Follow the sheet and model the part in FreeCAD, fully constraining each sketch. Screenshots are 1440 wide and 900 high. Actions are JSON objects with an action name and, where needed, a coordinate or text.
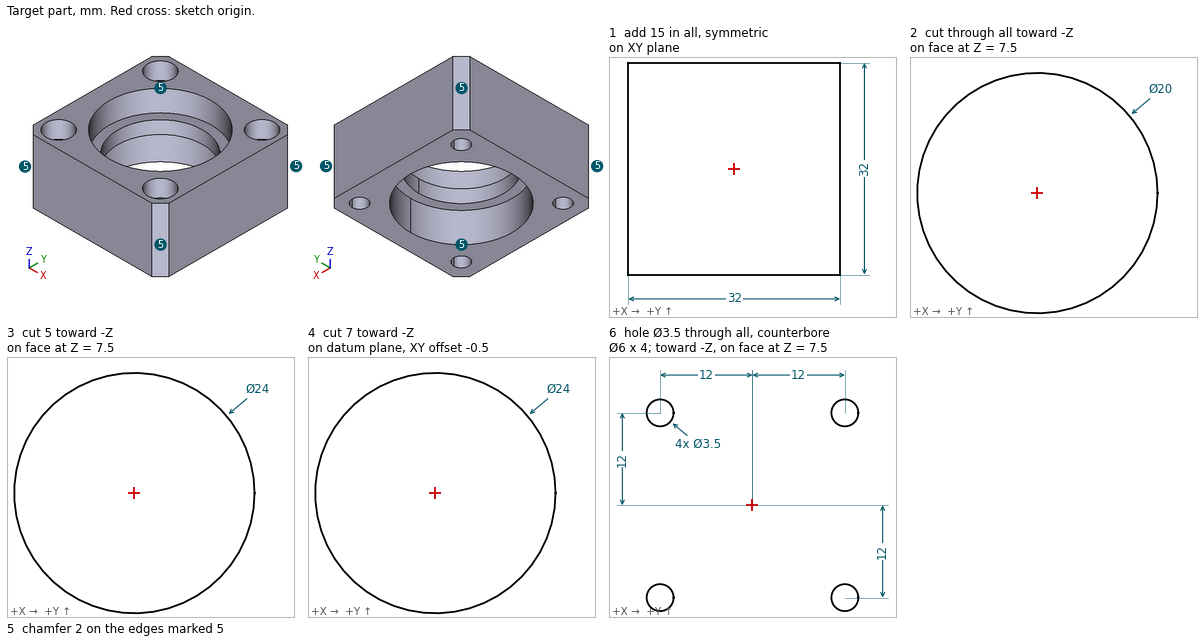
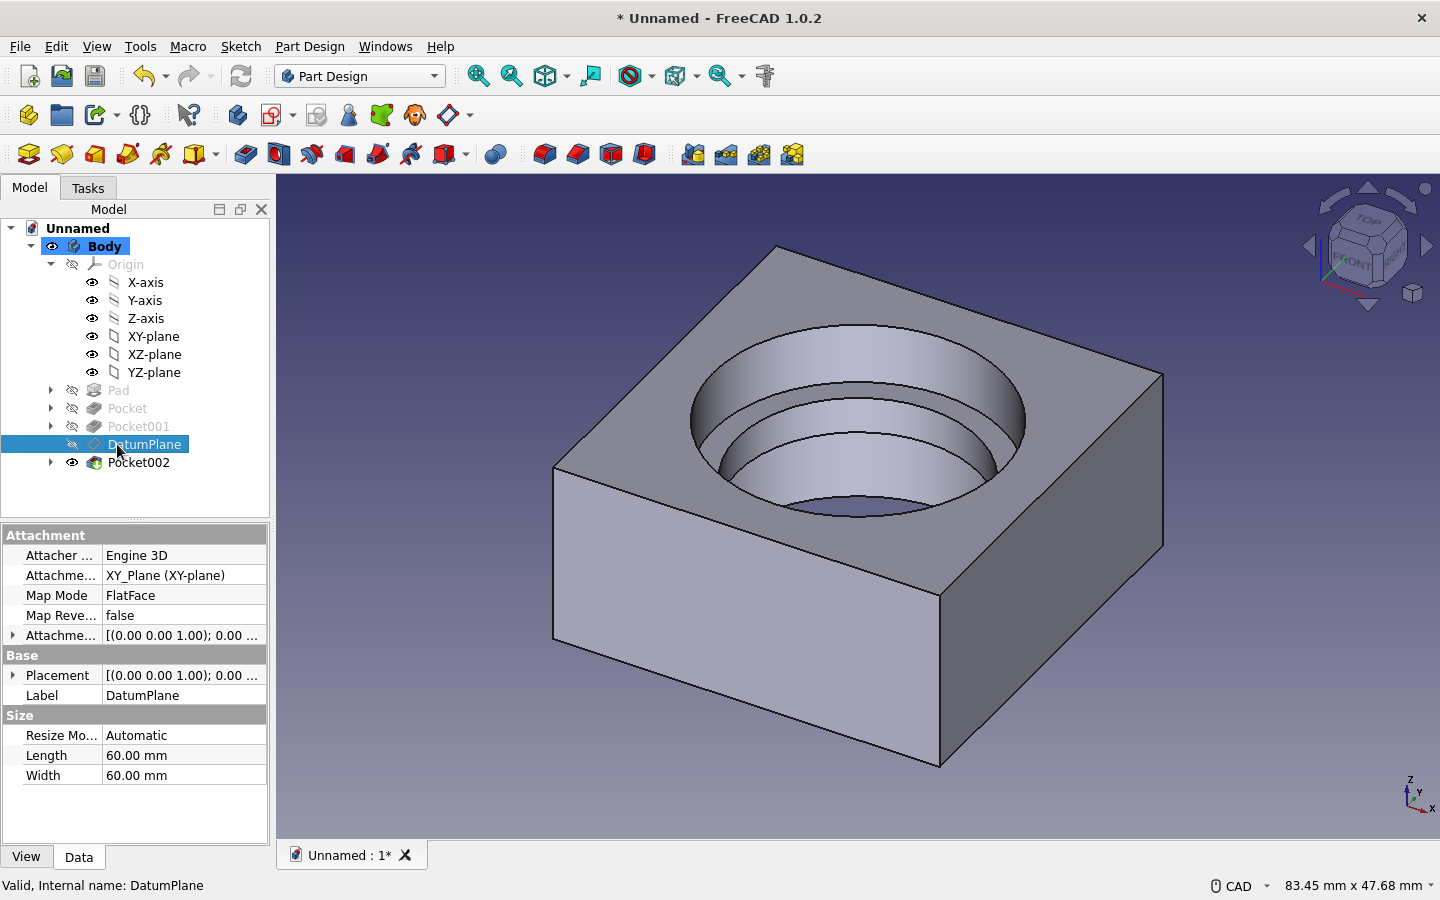
{"action": "left_click", "coordinate": [940, 680]}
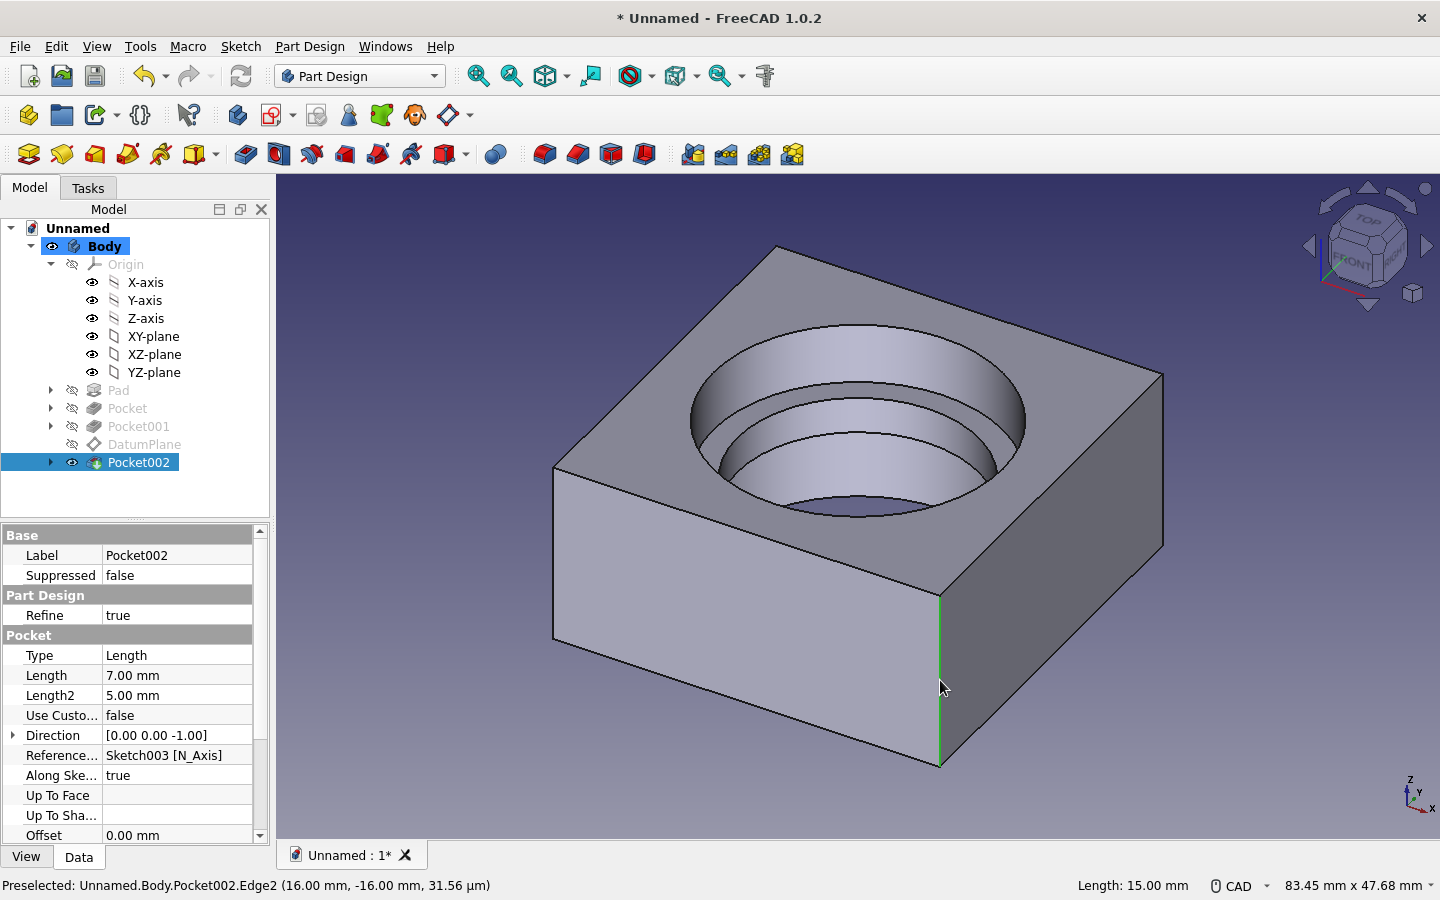
{"action": "key", "text": "0"}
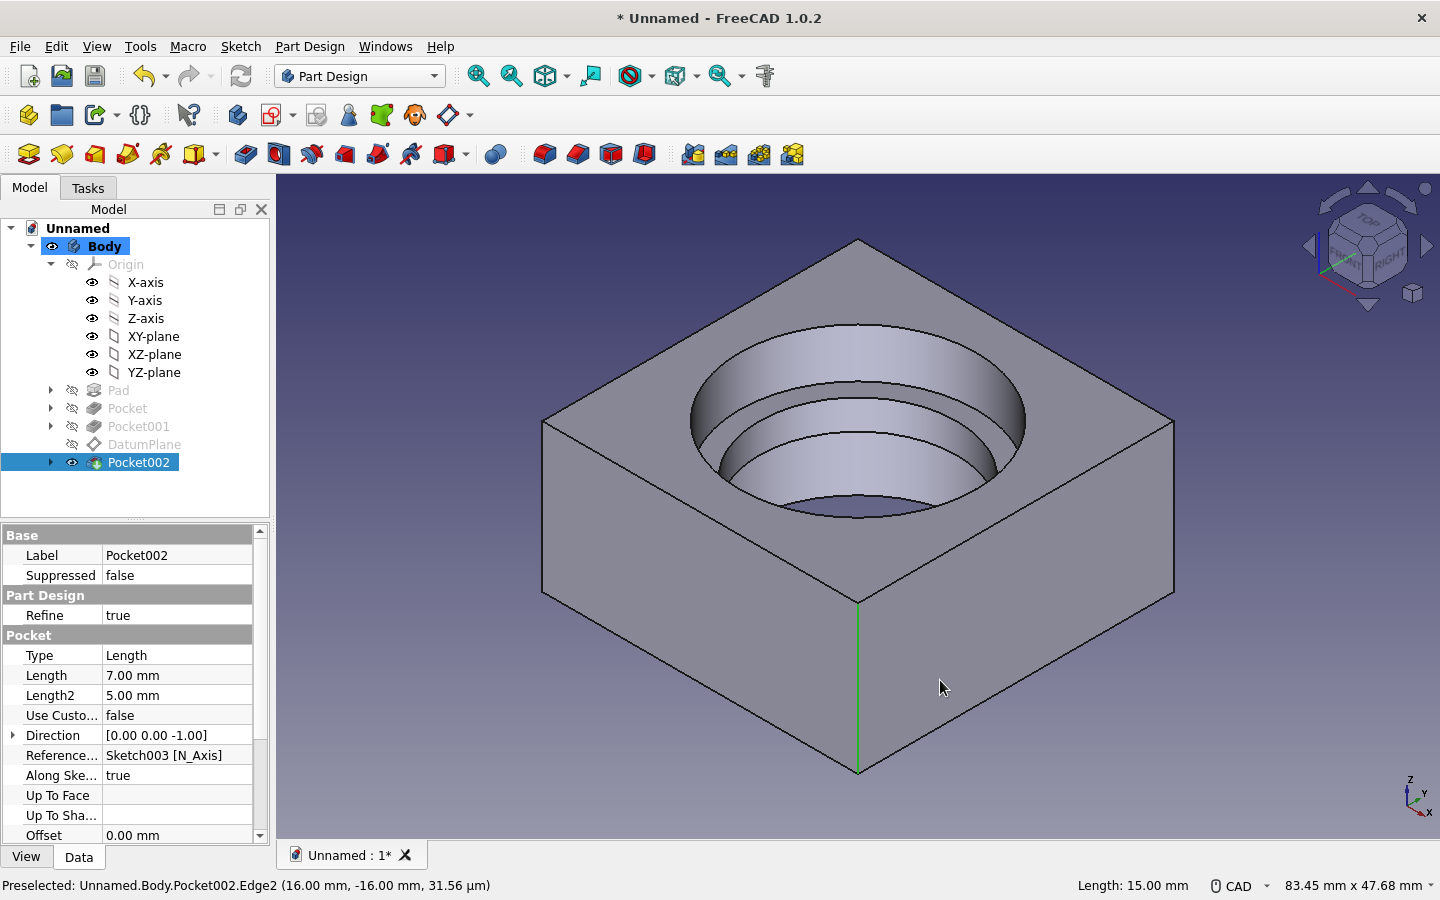
{"action": "key", "text": "2"}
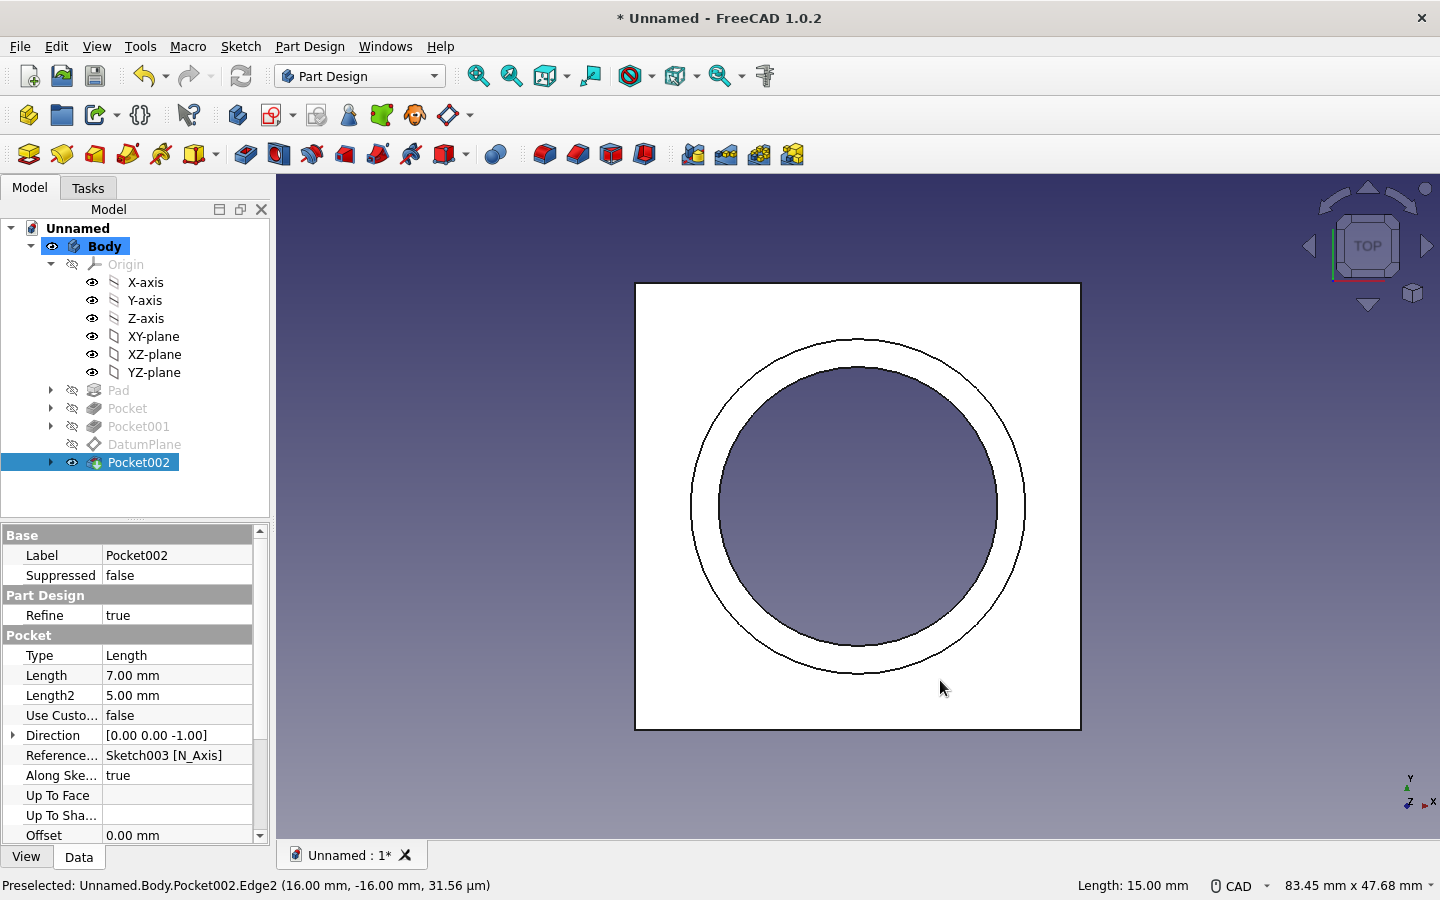
{"action": "key", "text": "1"}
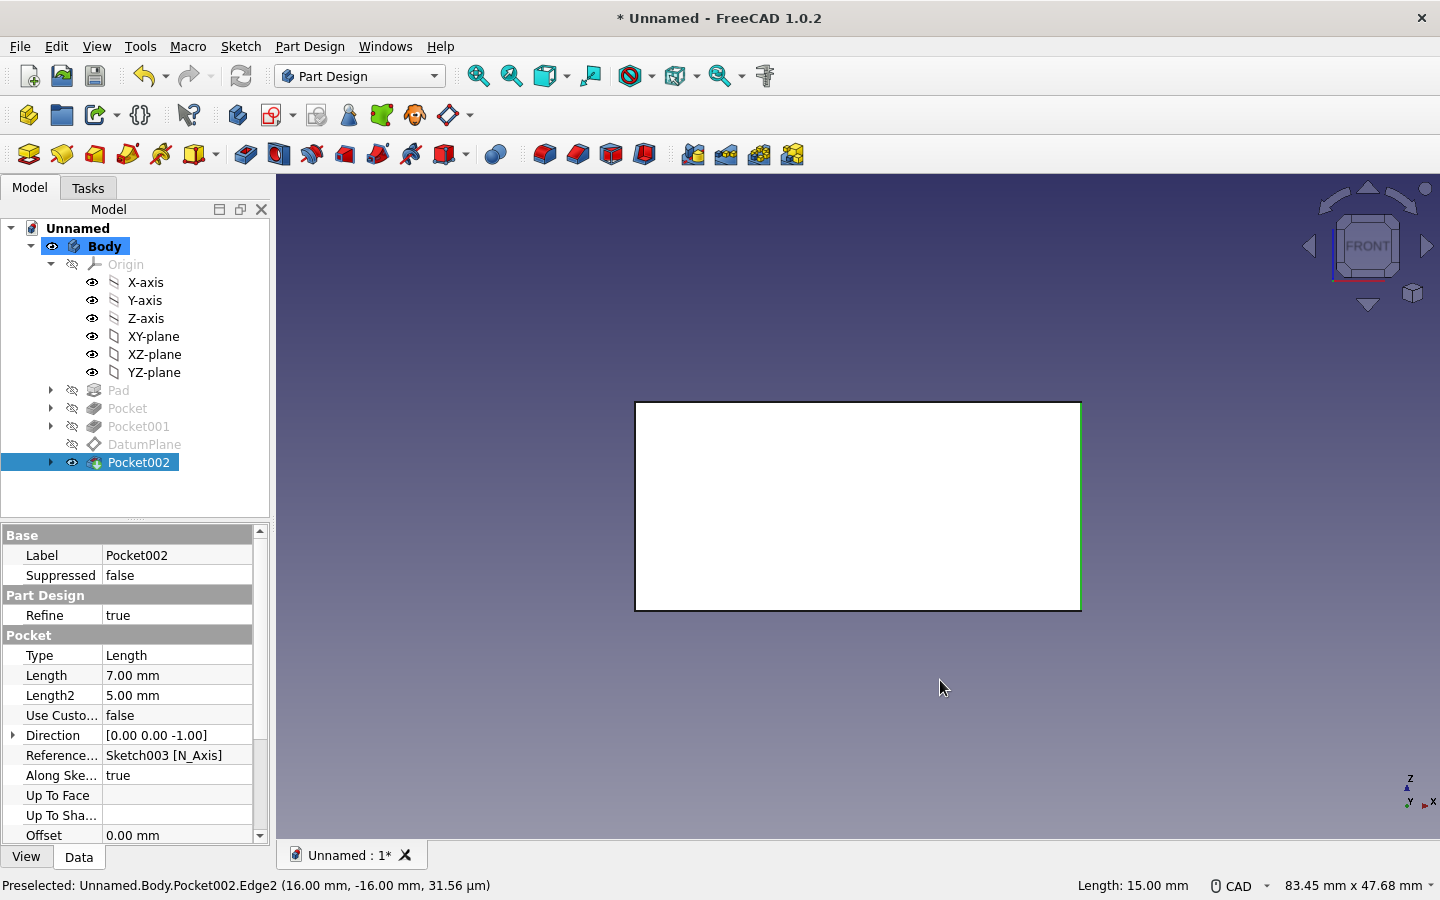
{"action": "key", "text": "v f"}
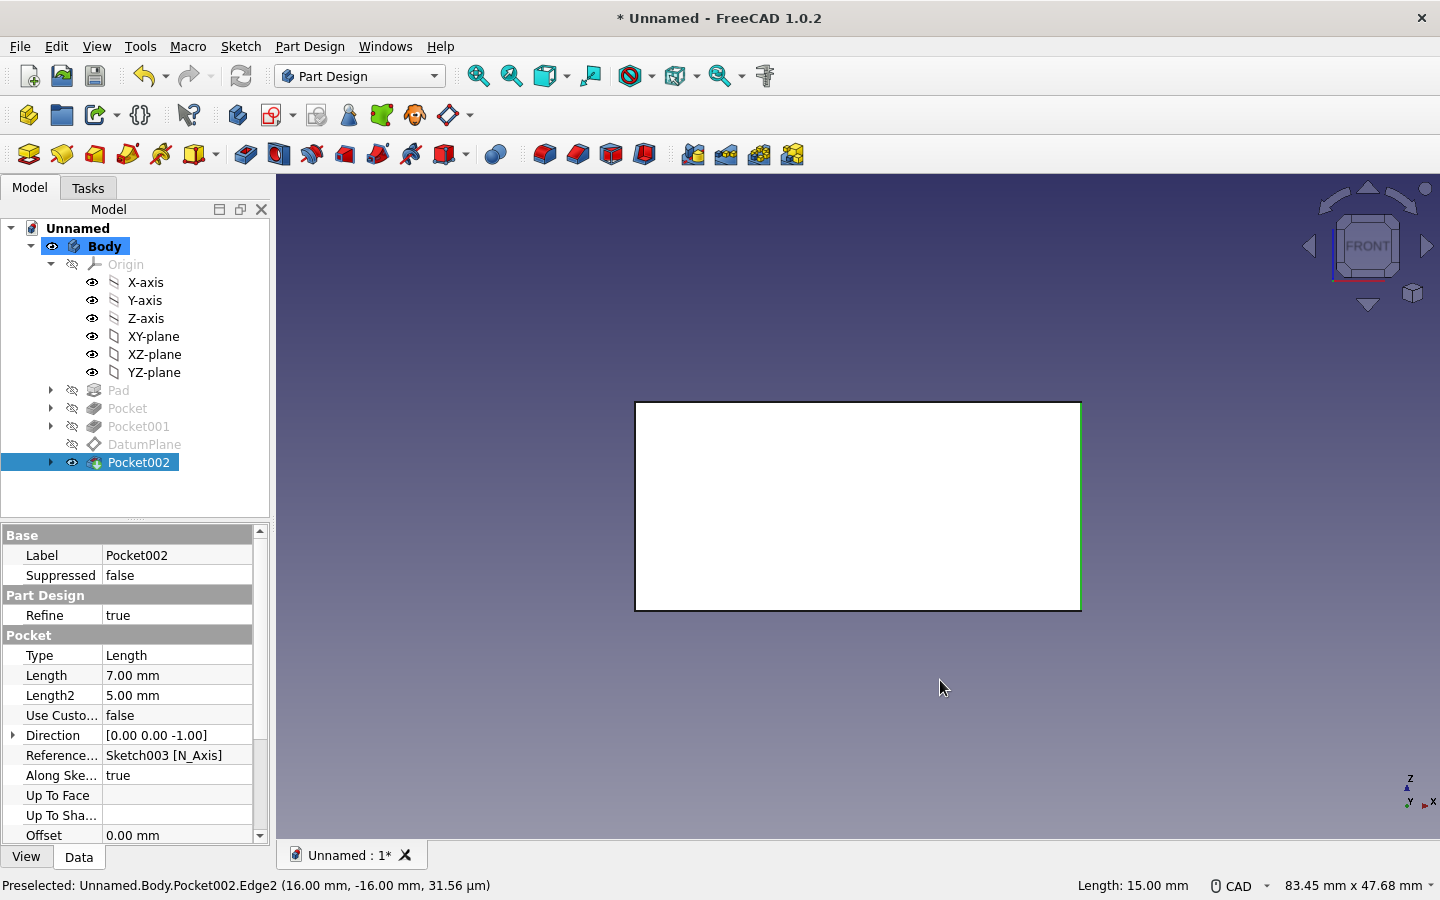
{"action": "left_click", "coordinate": [635, 506], "text": "ctrl"}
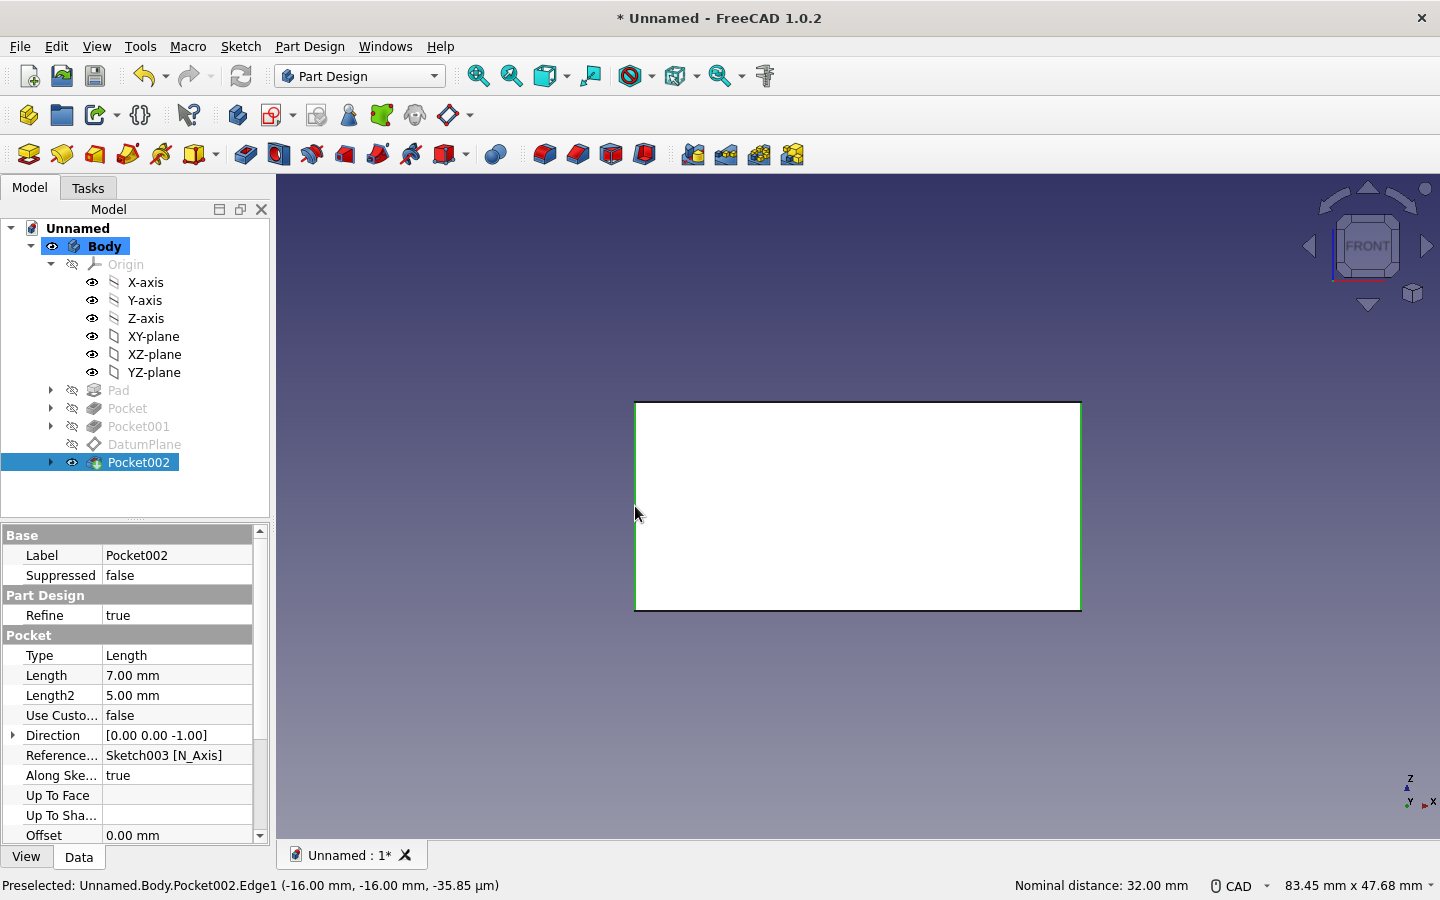
{"action": "key", "text": "3"}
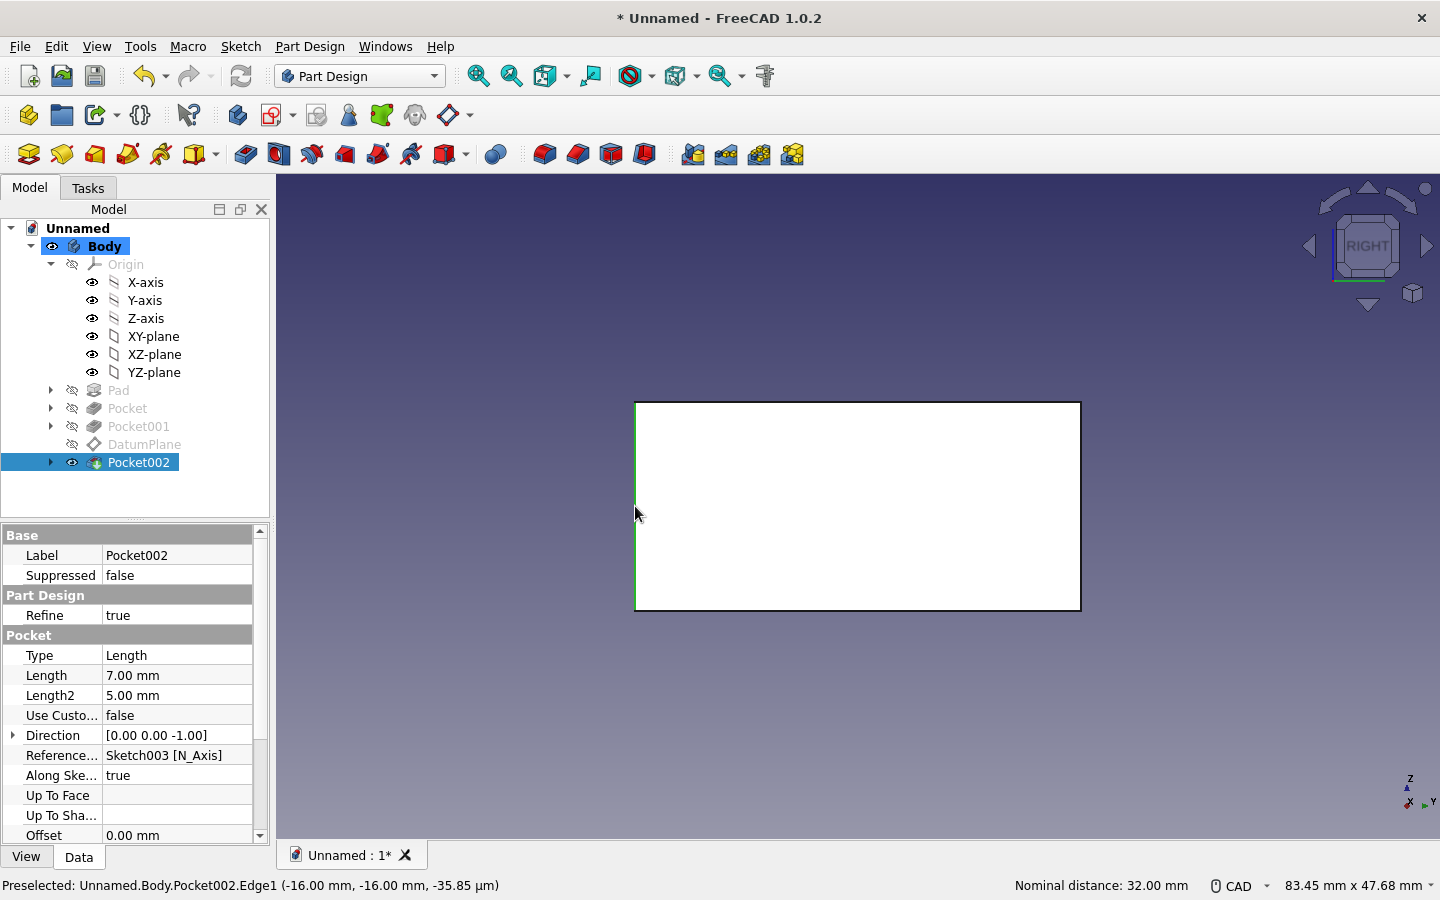
{"action": "left_click", "coordinate": [479, 76]}